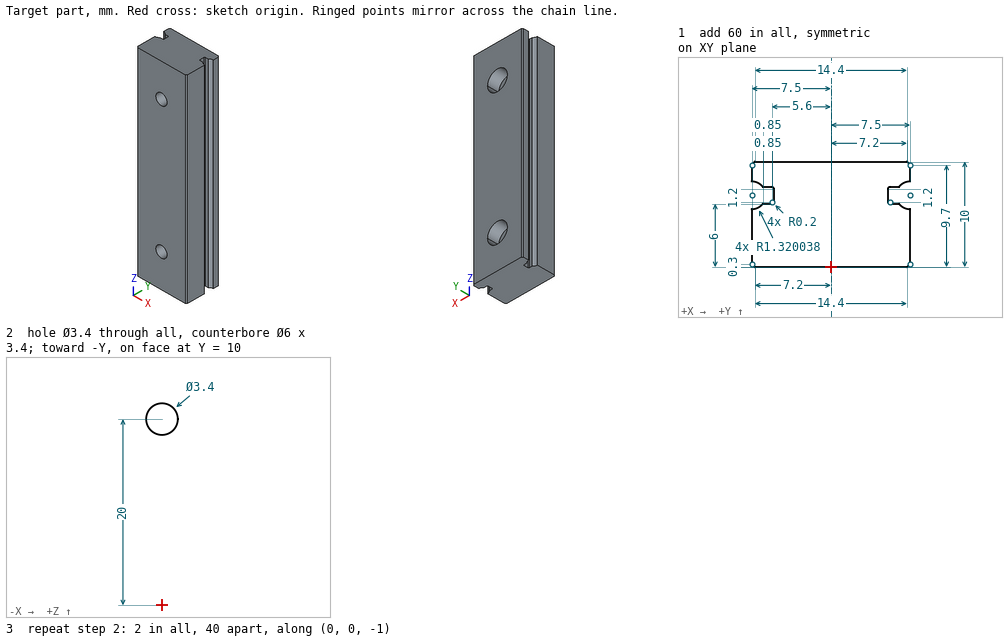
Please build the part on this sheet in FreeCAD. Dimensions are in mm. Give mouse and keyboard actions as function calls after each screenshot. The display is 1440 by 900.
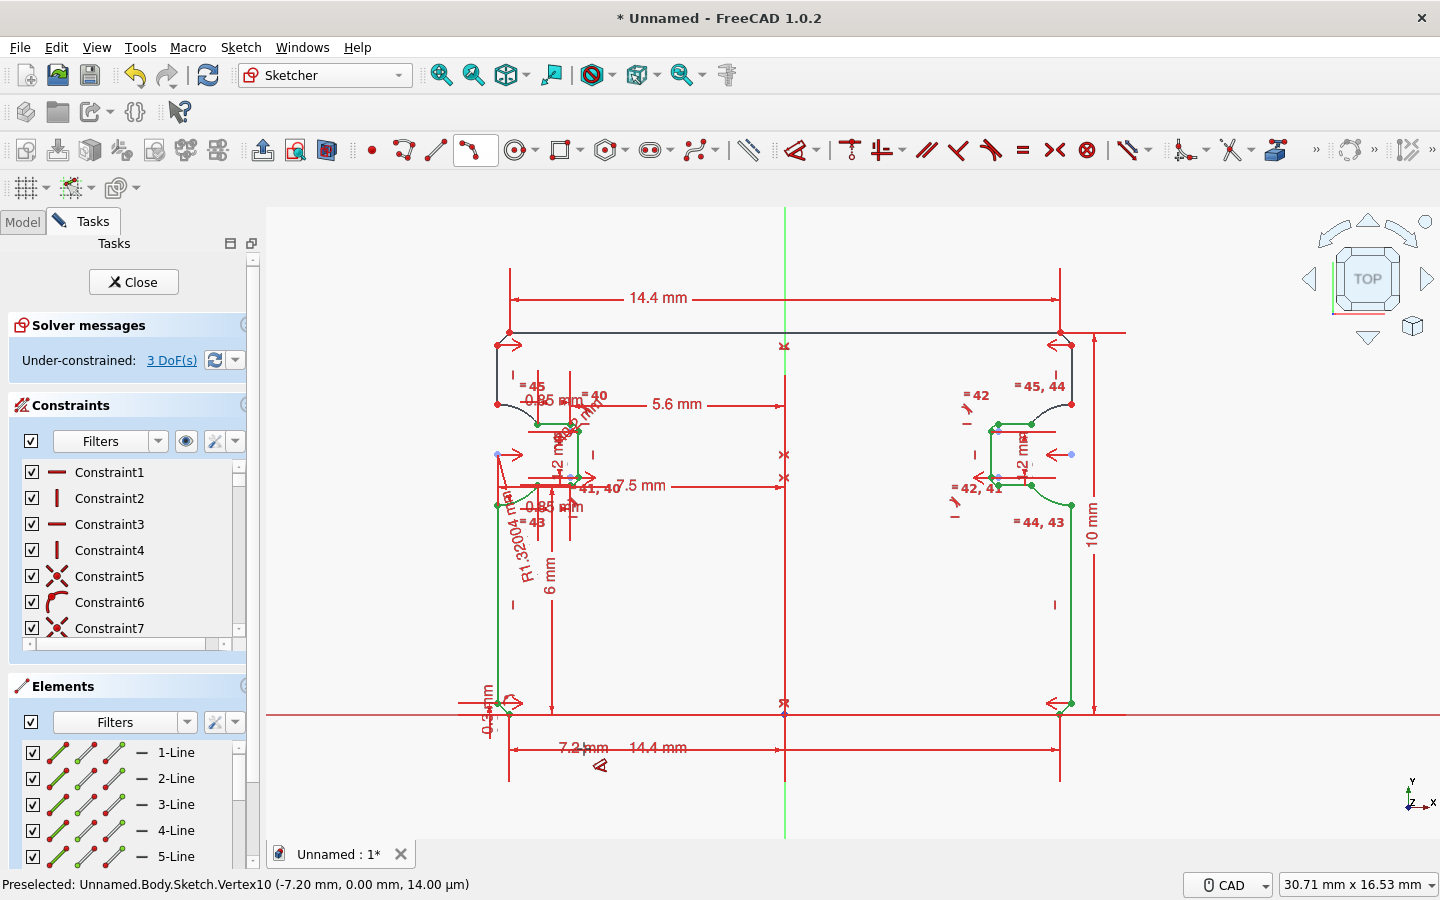
click(1072, 404)
click(928, 749)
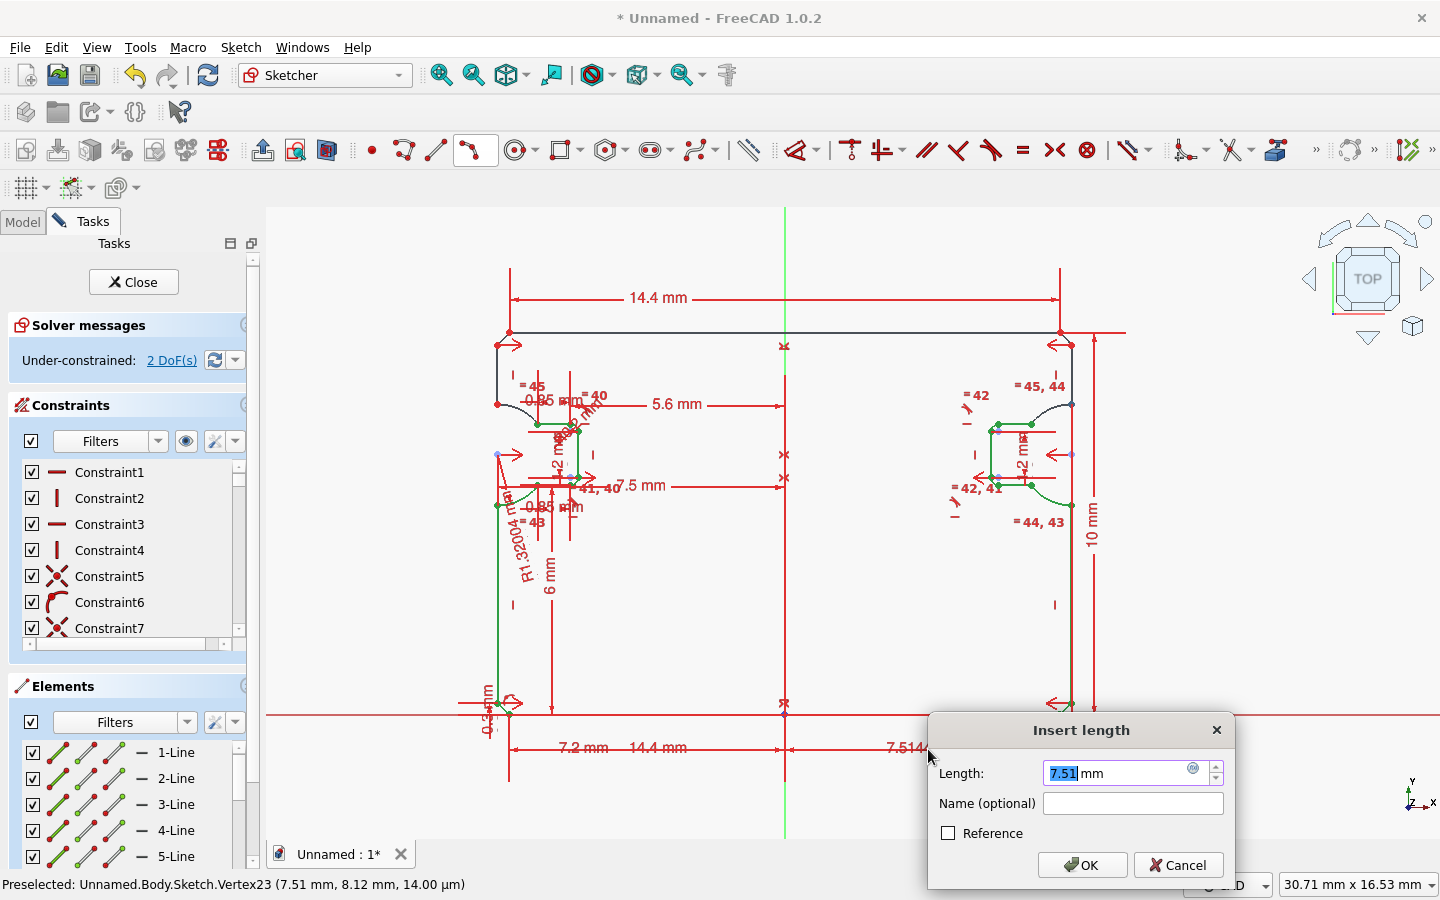
text(7.5)
key(Return)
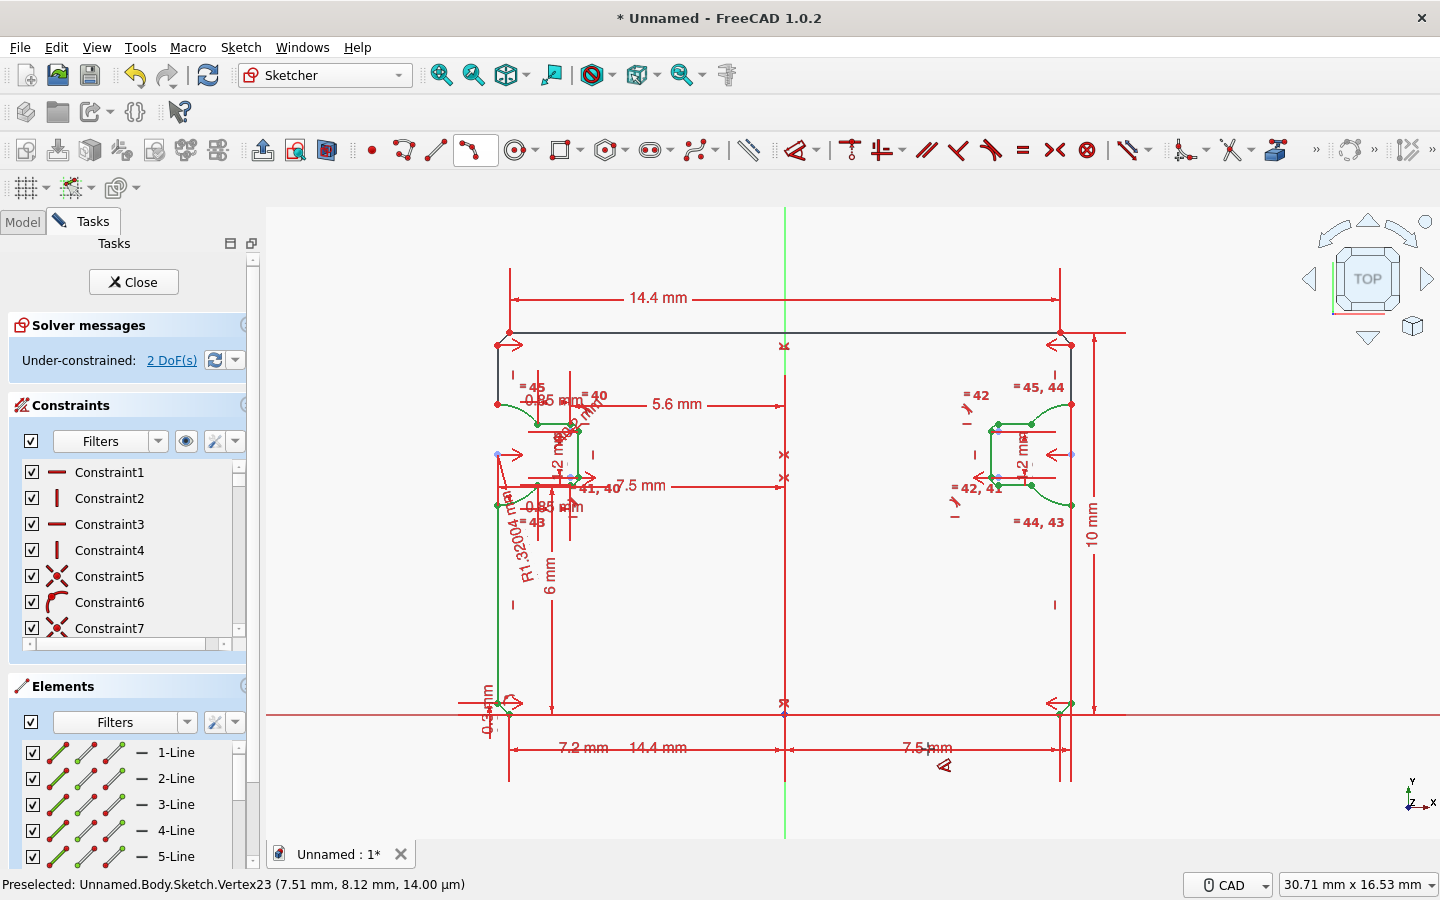
click(1071, 345)
click(1105, 445)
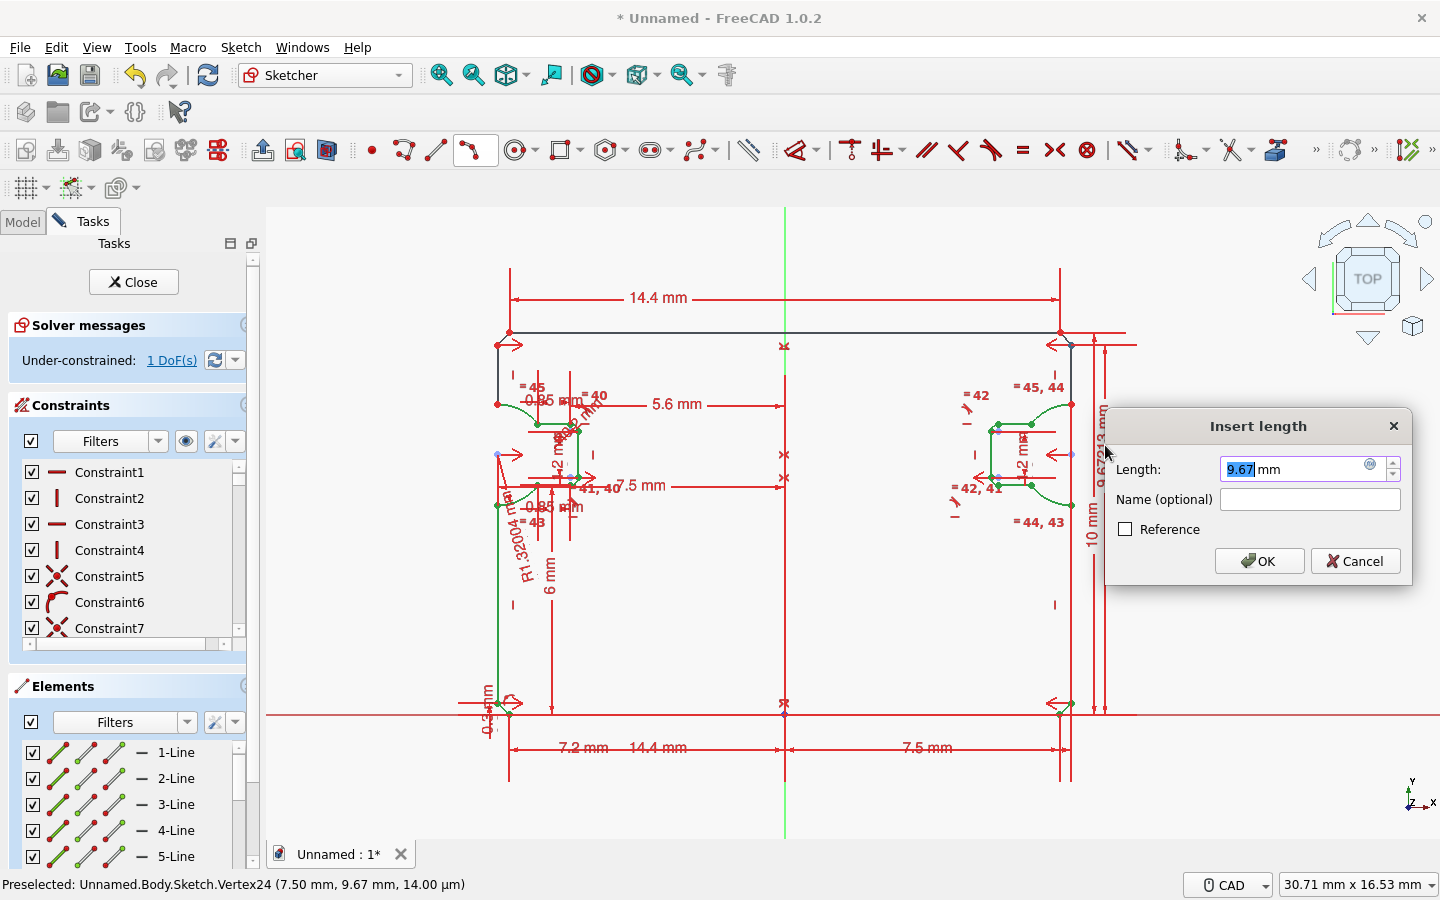
text(9.7)
key(Return)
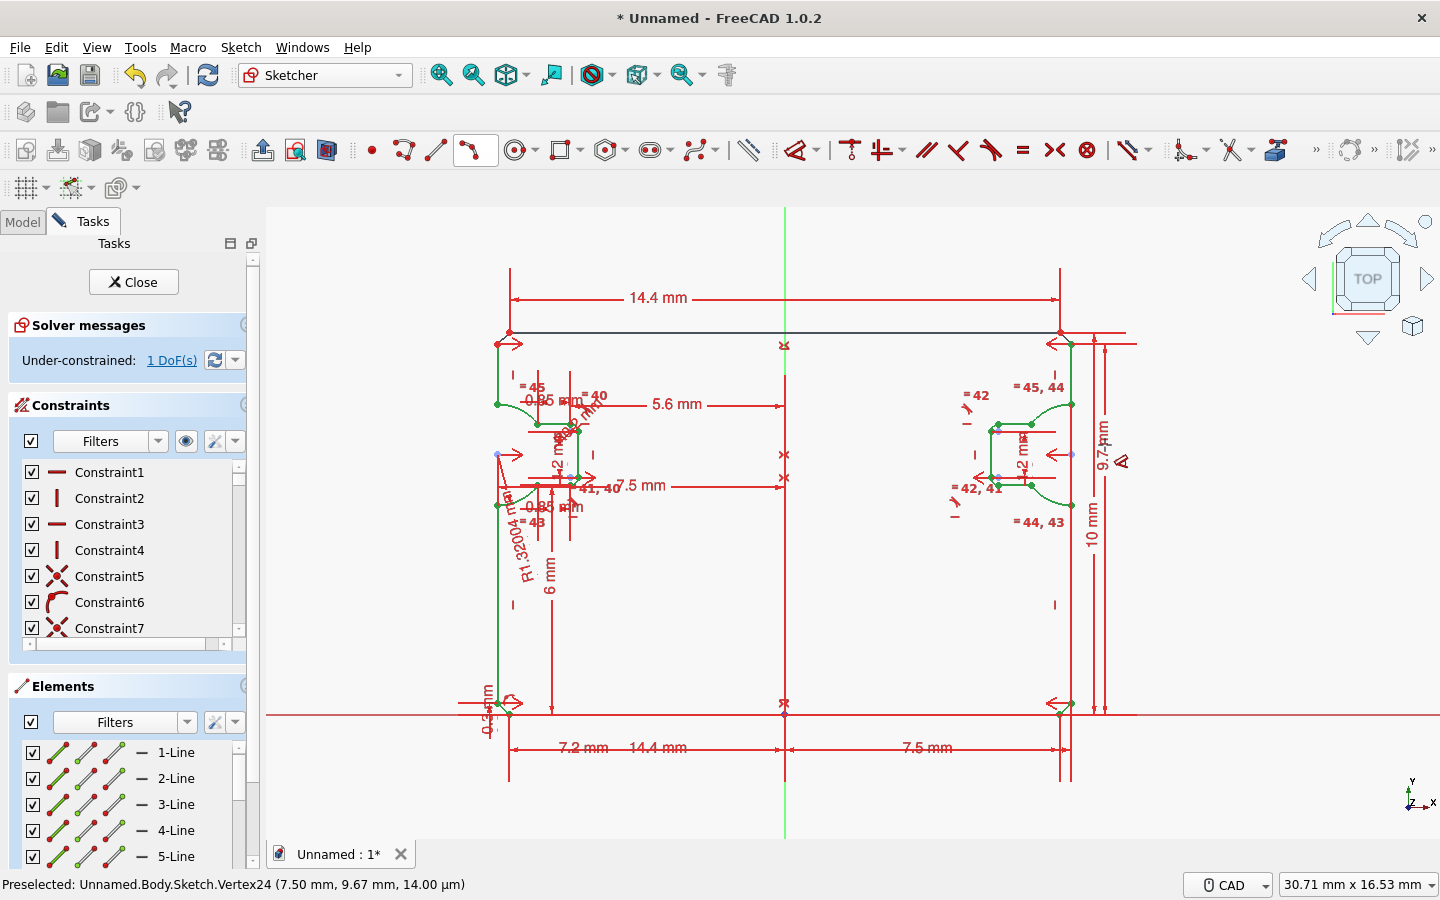
click(1060, 333)
click(826, 749)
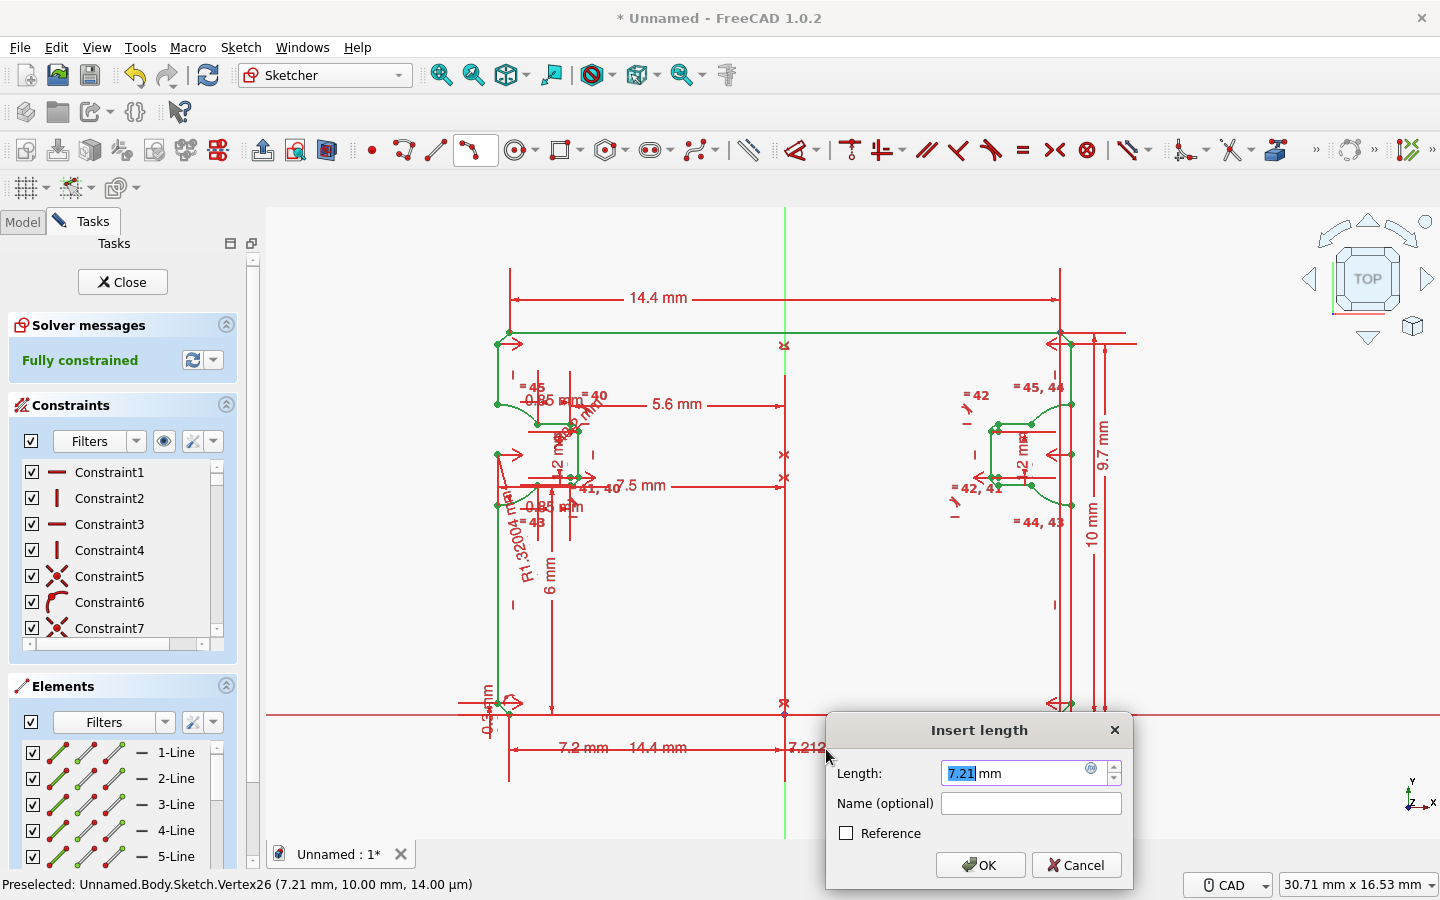
text(7.2)
key(Return)
key(Escape)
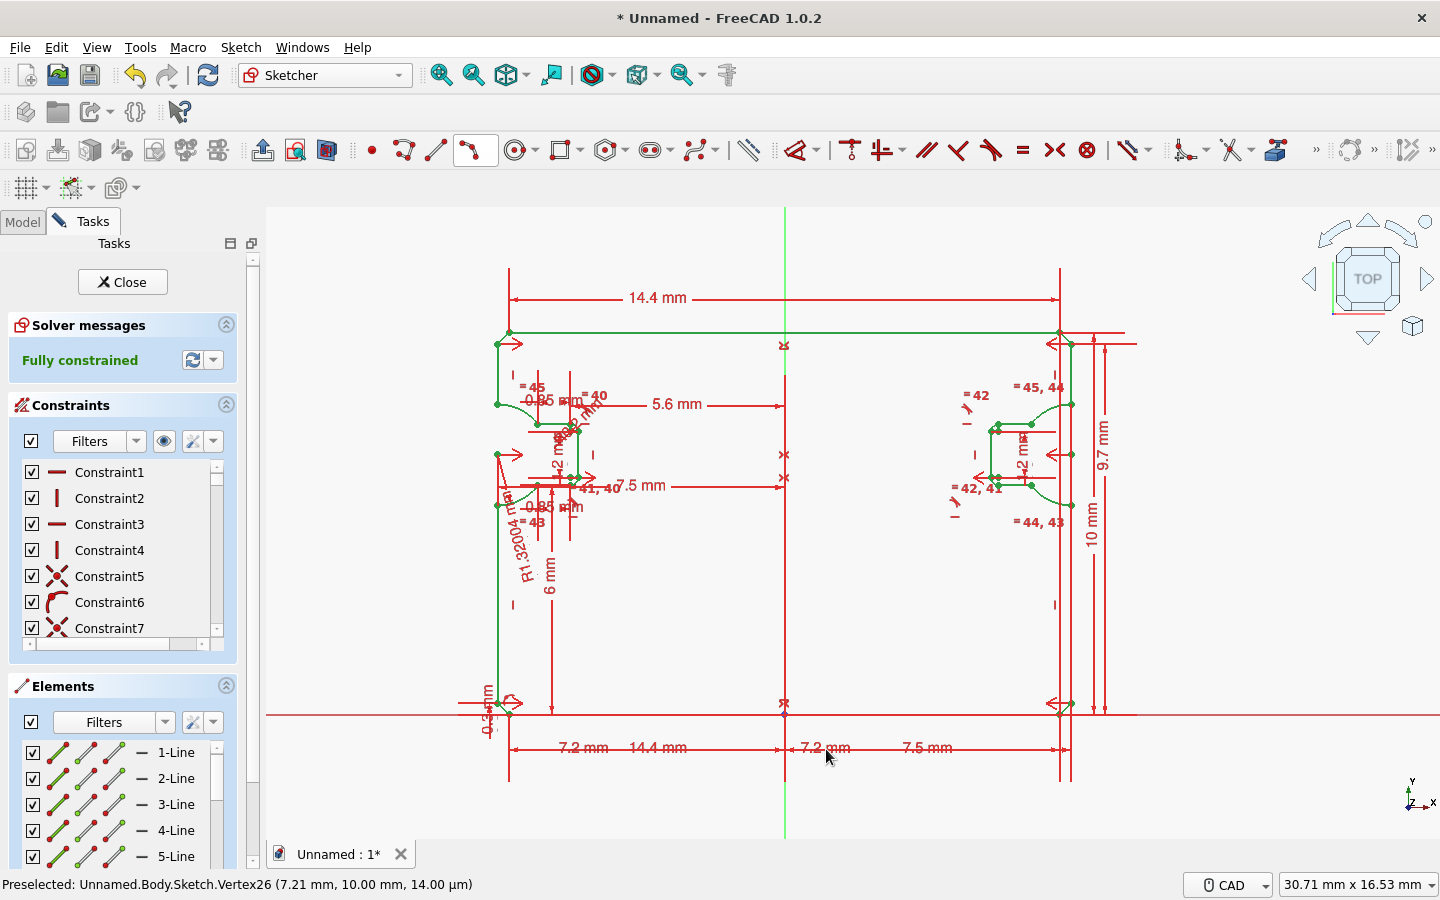
click(123, 282)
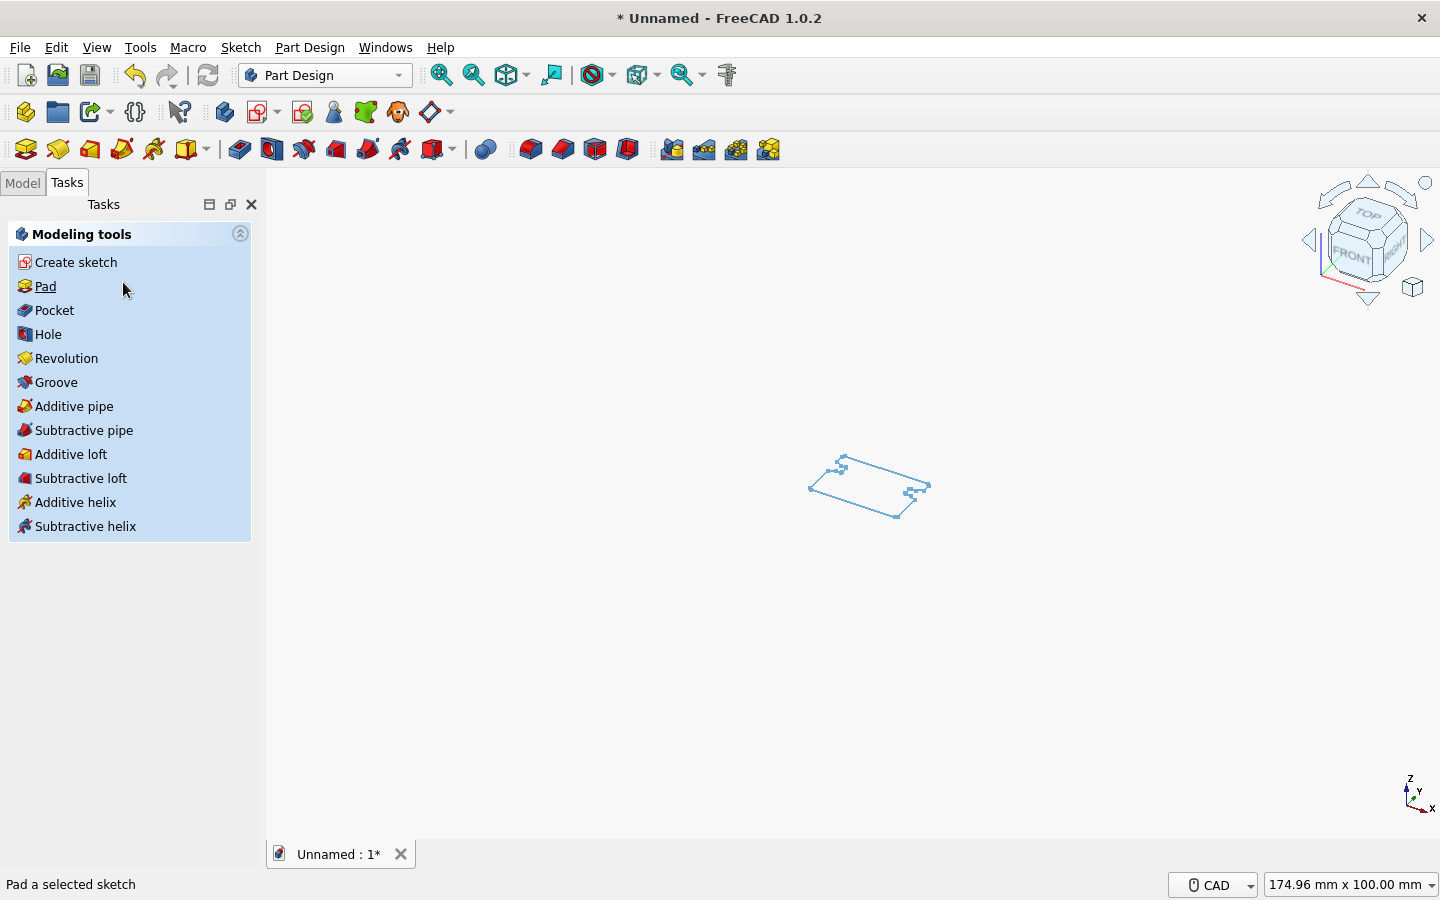
click(26, 150)